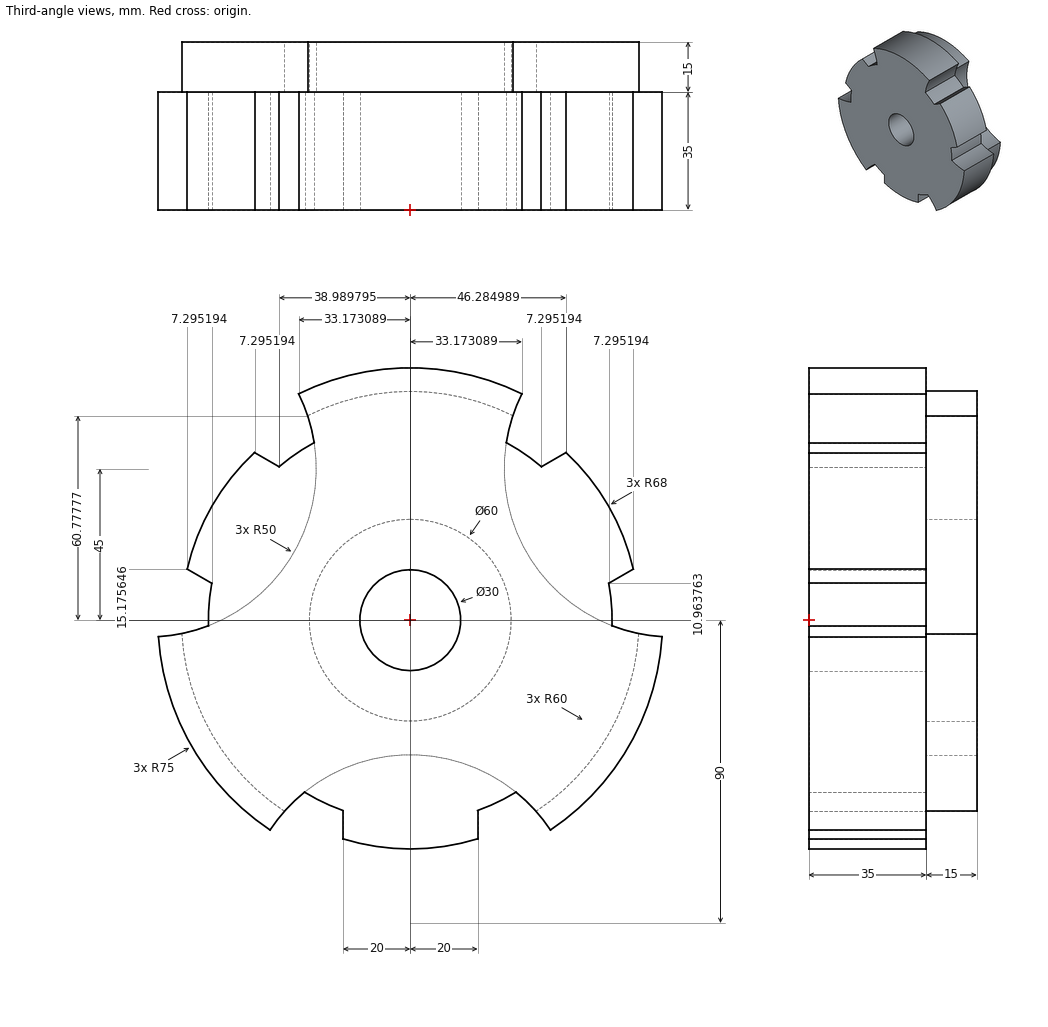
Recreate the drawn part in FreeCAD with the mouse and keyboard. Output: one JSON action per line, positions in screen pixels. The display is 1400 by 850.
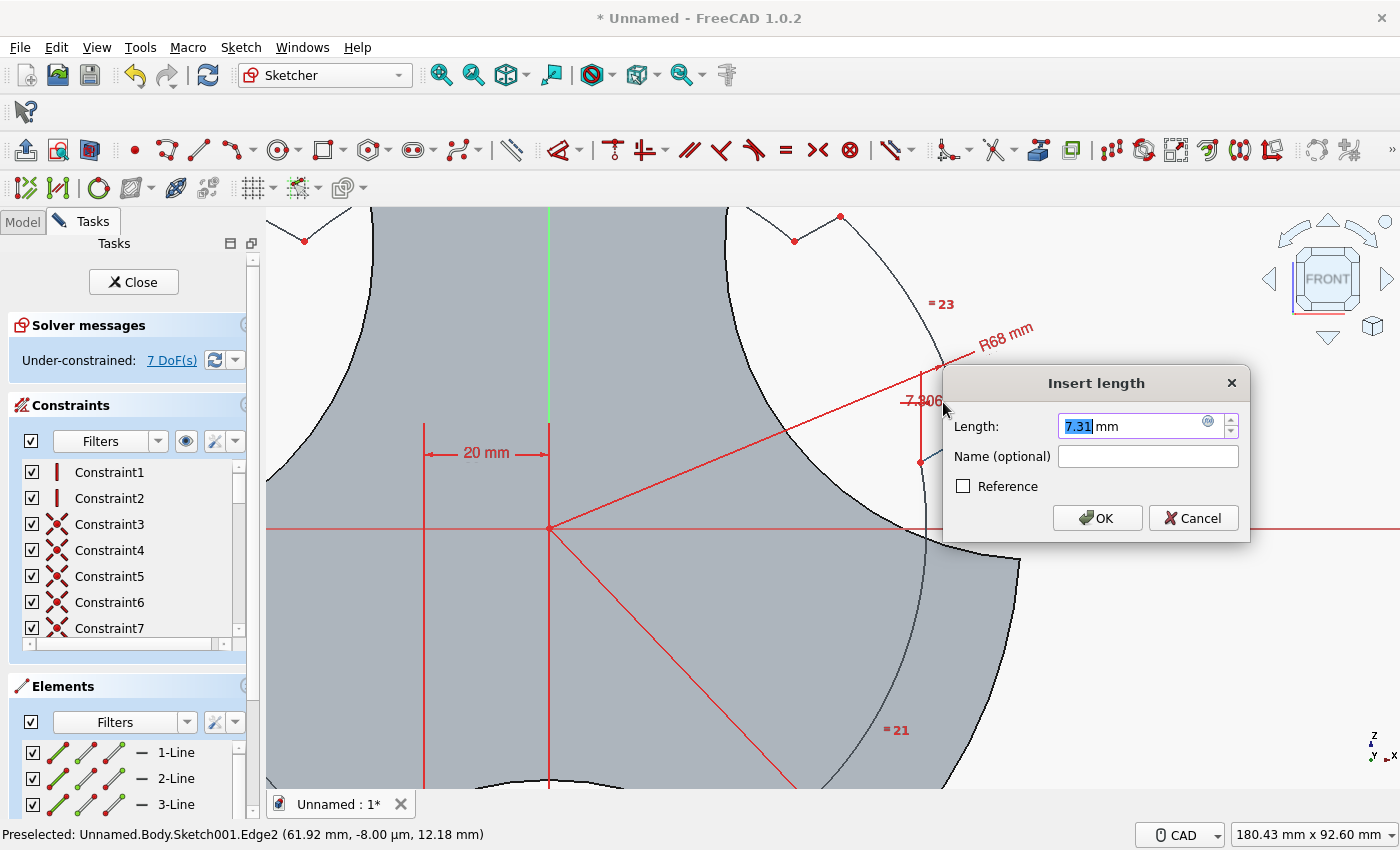
{"action": "type", "text": "7.295194"}
{"action": "key", "text": "Return"}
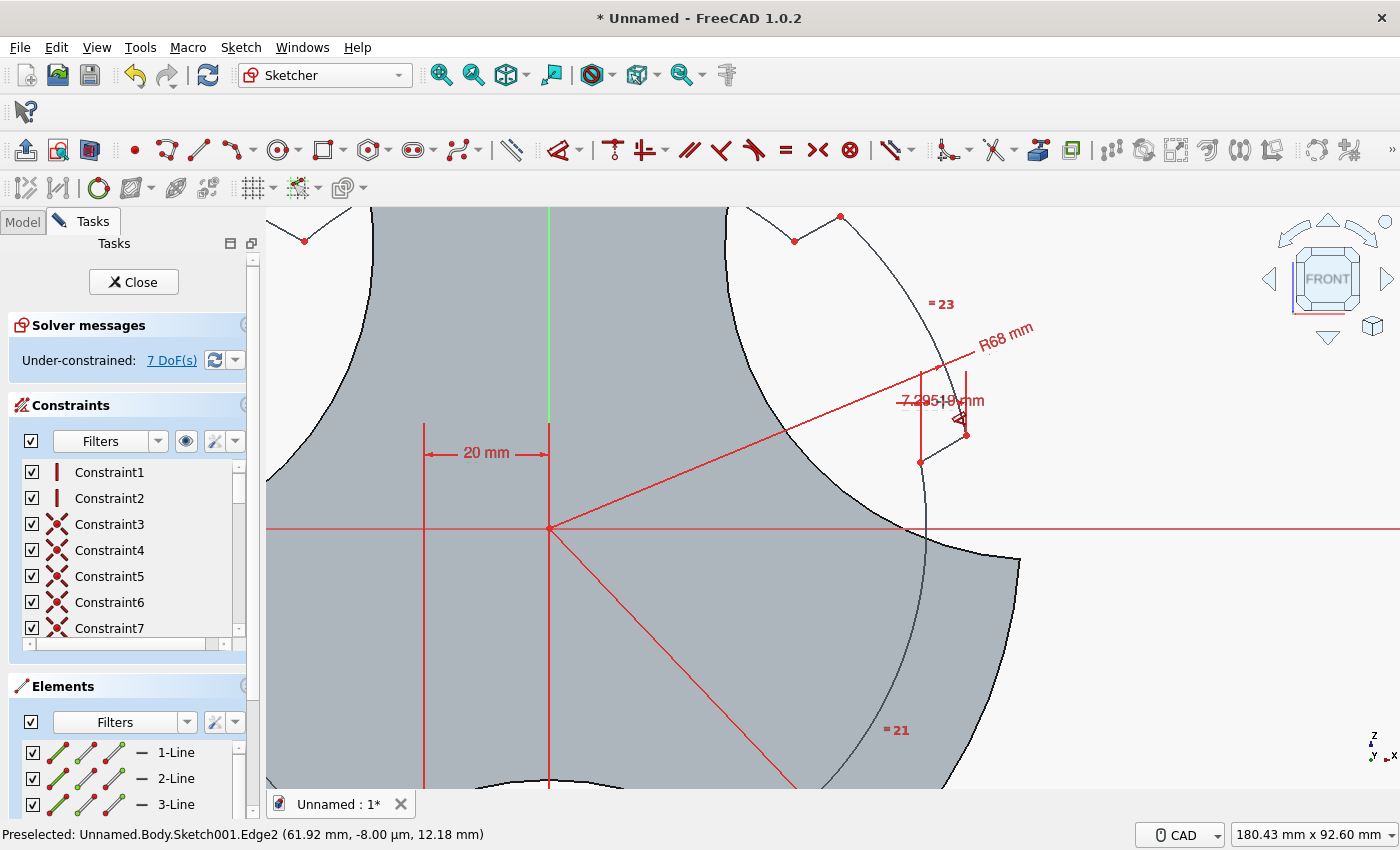
{"action": "scroll", "coordinate": [804, 237], "scroll_direction": "up", "scroll_amount": 2}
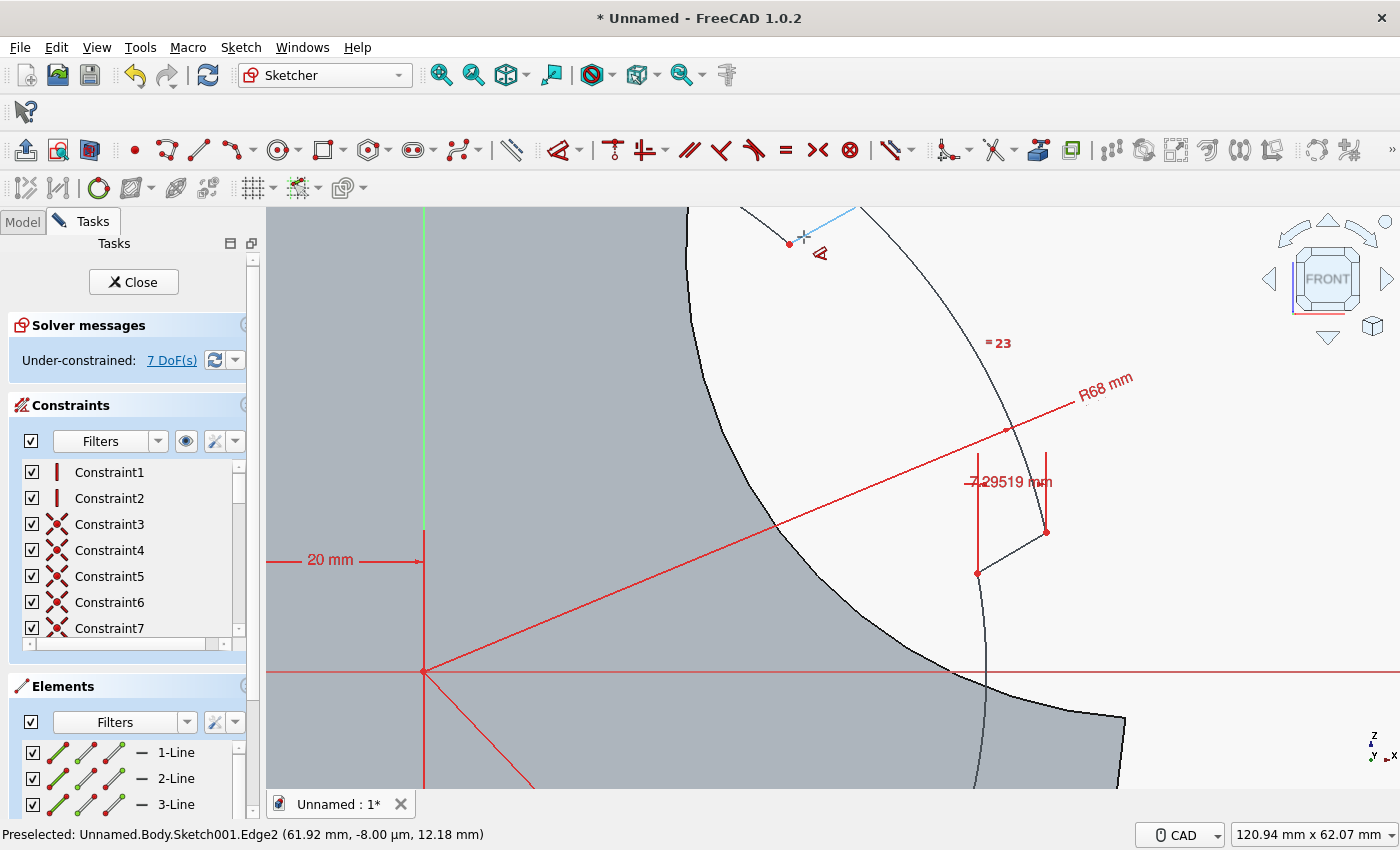
{"action": "left_click", "coordinate": [803, 237]}
{"action": "left_click", "coordinate": [824, 278]}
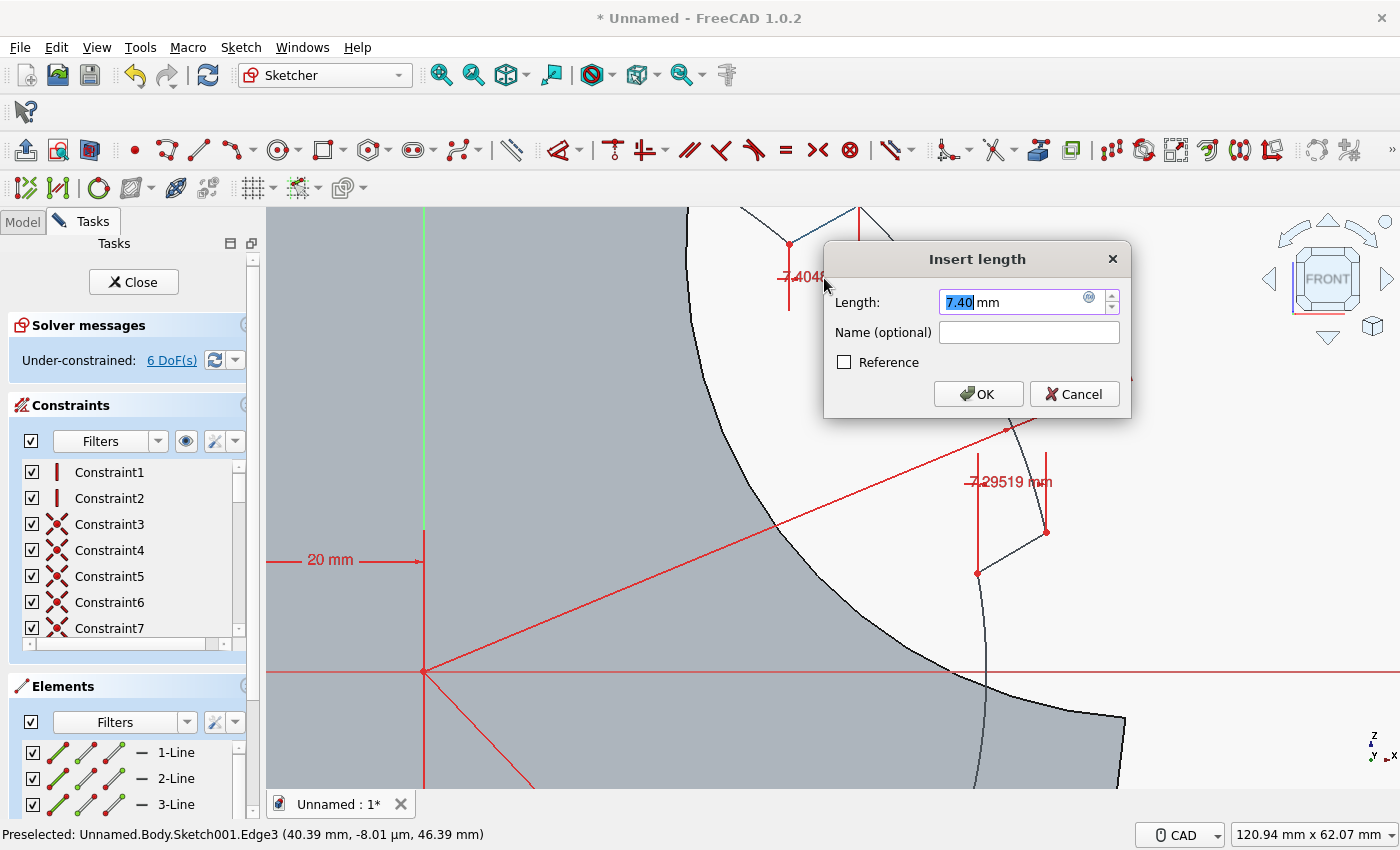
{"action": "type", "text": "7.295194"}
{"action": "key", "text": "Return"}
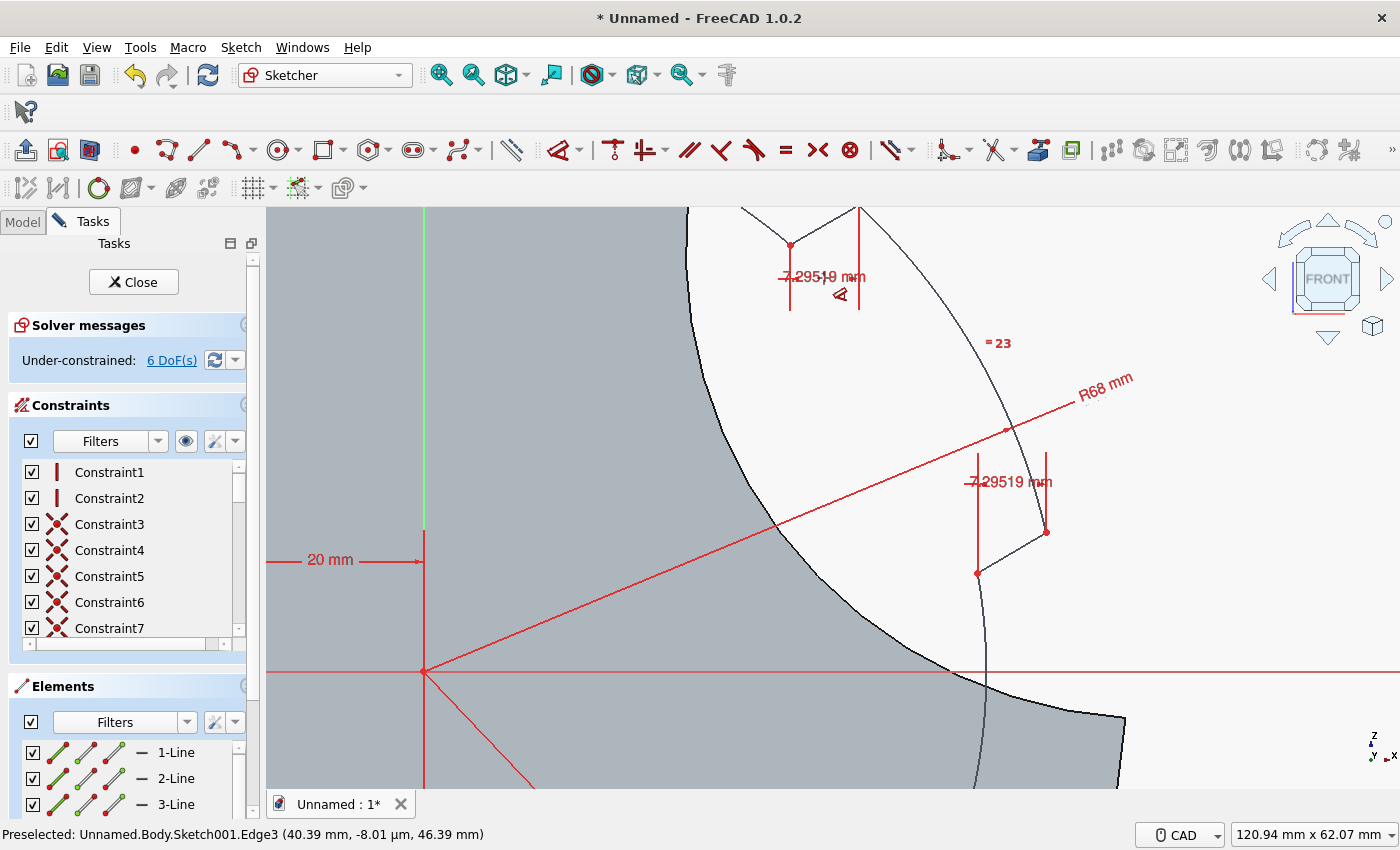
{"action": "scroll", "coordinate": [911, 407], "scroll_direction": "down", "scroll_amount": 6}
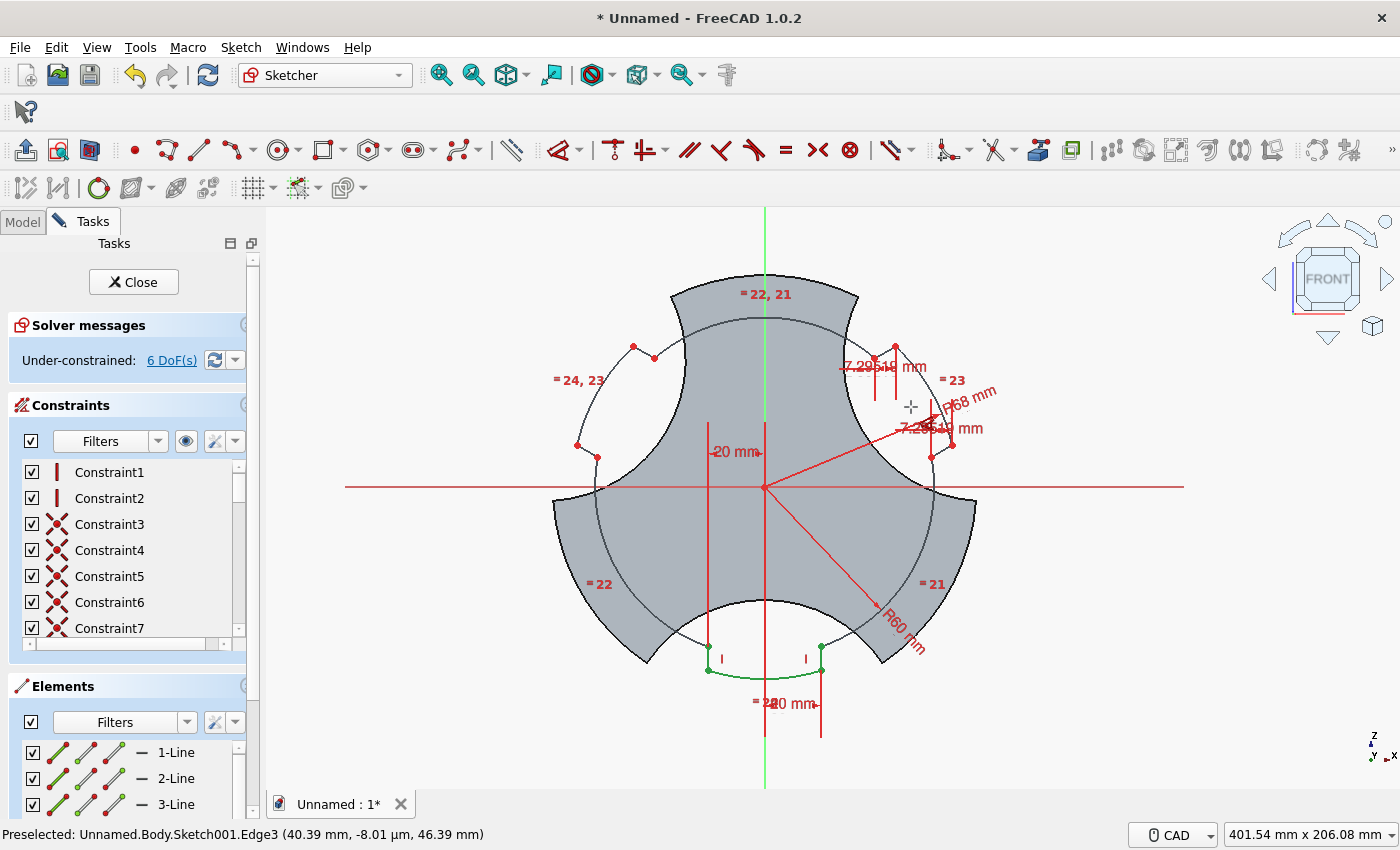
{"action": "scroll", "coordinate": [648, 355], "scroll_direction": "up", "scroll_amount": 4}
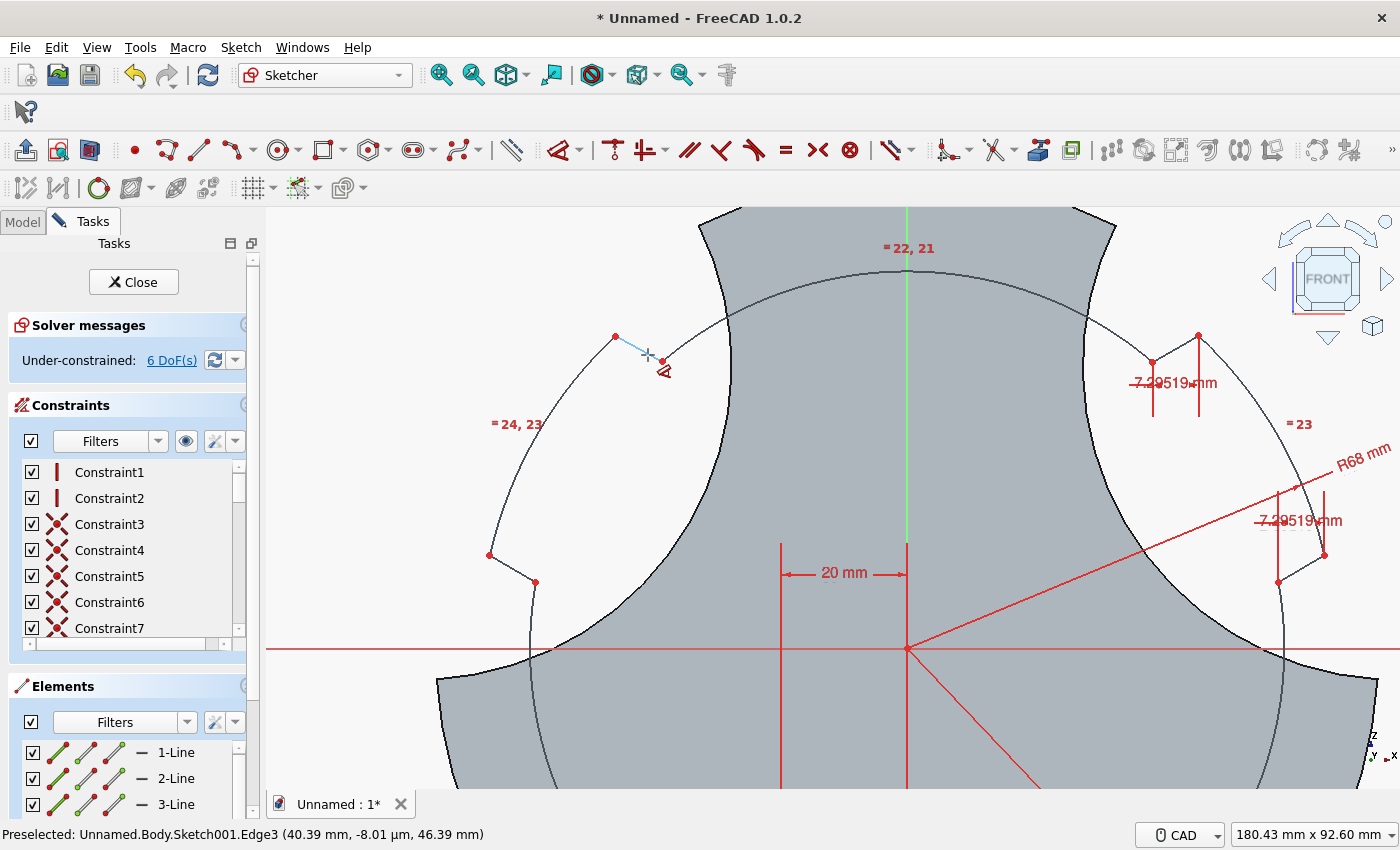
{"action": "left_click", "coordinate": [648, 354]}
{"action": "left_click", "coordinate": [639, 302]}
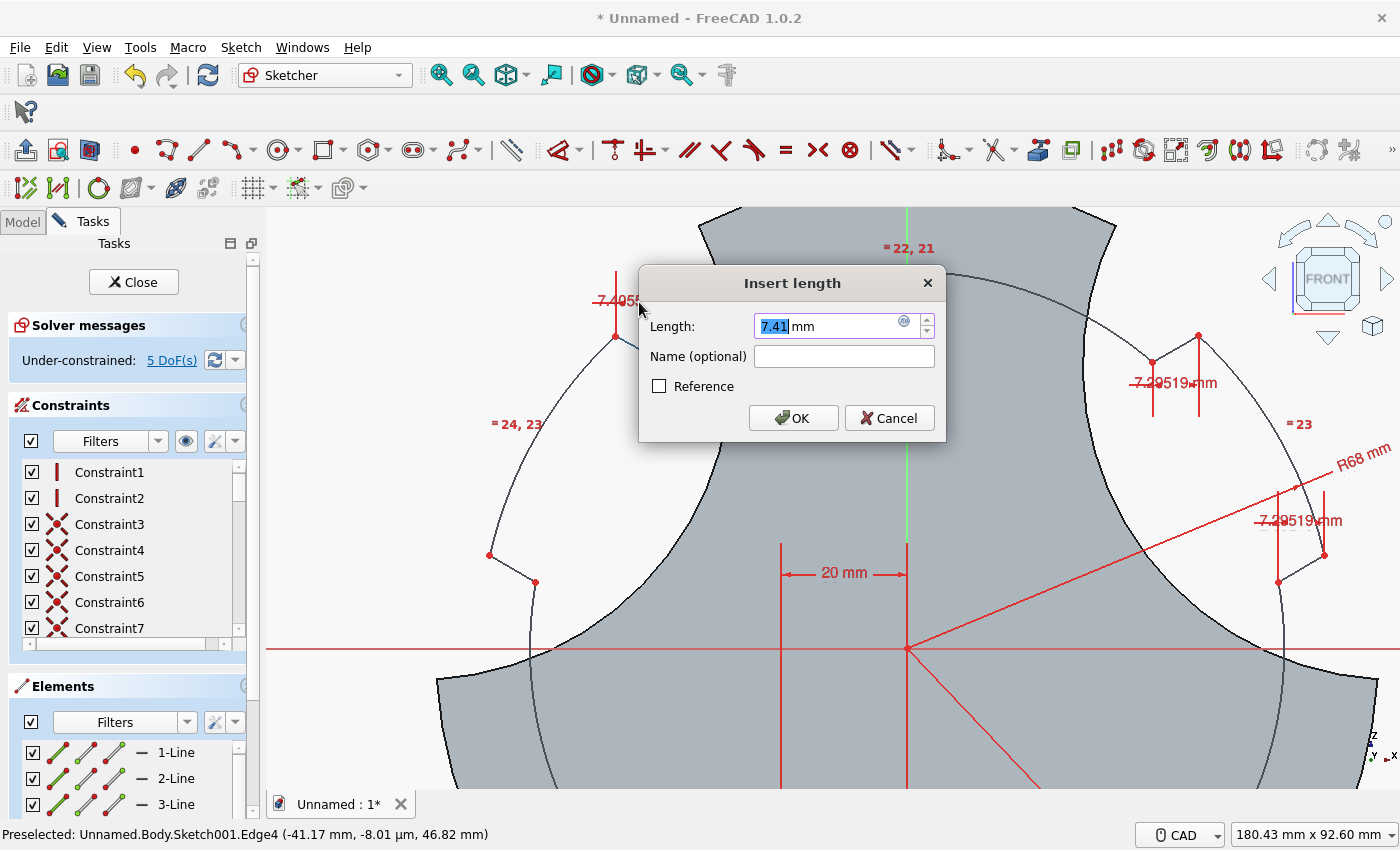
{"action": "type", "text": "7.295194"}
{"action": "key", "text": "Return"}